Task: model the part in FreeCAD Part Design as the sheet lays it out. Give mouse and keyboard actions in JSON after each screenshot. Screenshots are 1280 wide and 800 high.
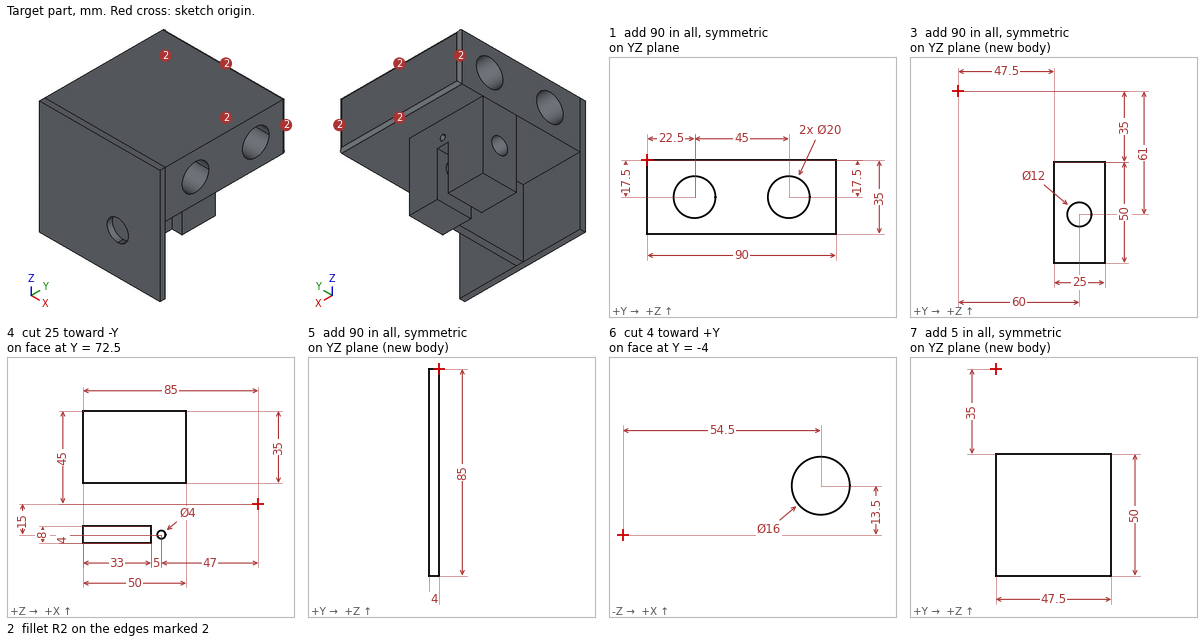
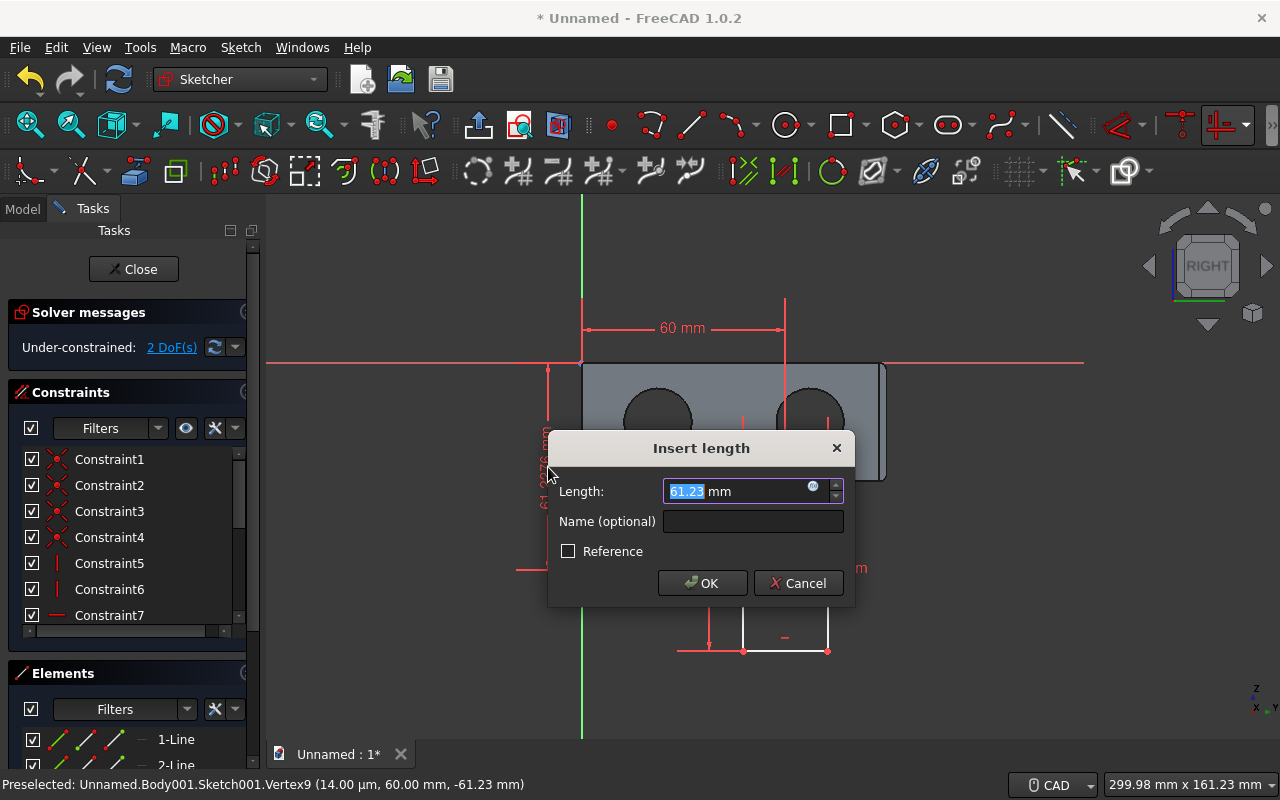
{"action": "type", "text": "61"}
{"action": "key", "text": "Return"}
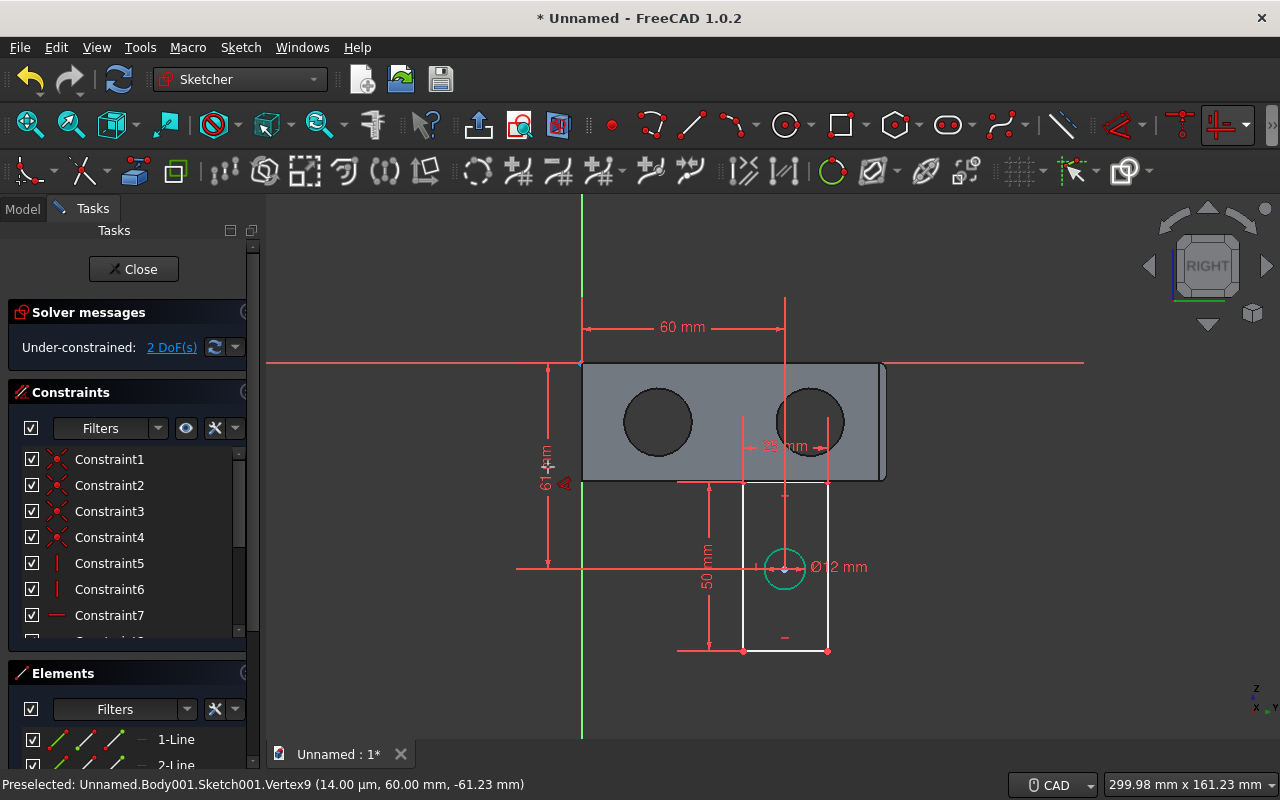
{"action": "left_click", "coordinate": [743, 482]}
{"action": "left_click", "coordinate": [548, 423]}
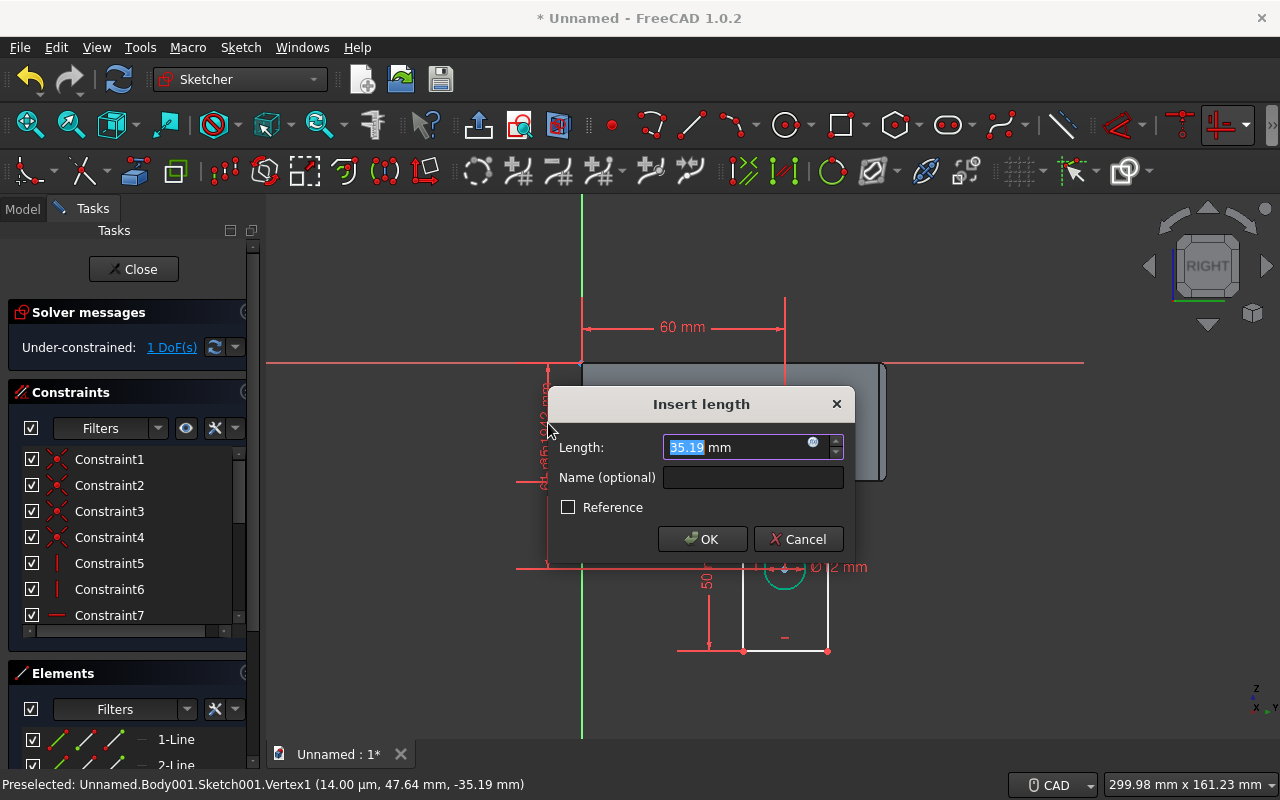
{"action": "type", "text": "35"}
{"action": "key", "text": "Return"}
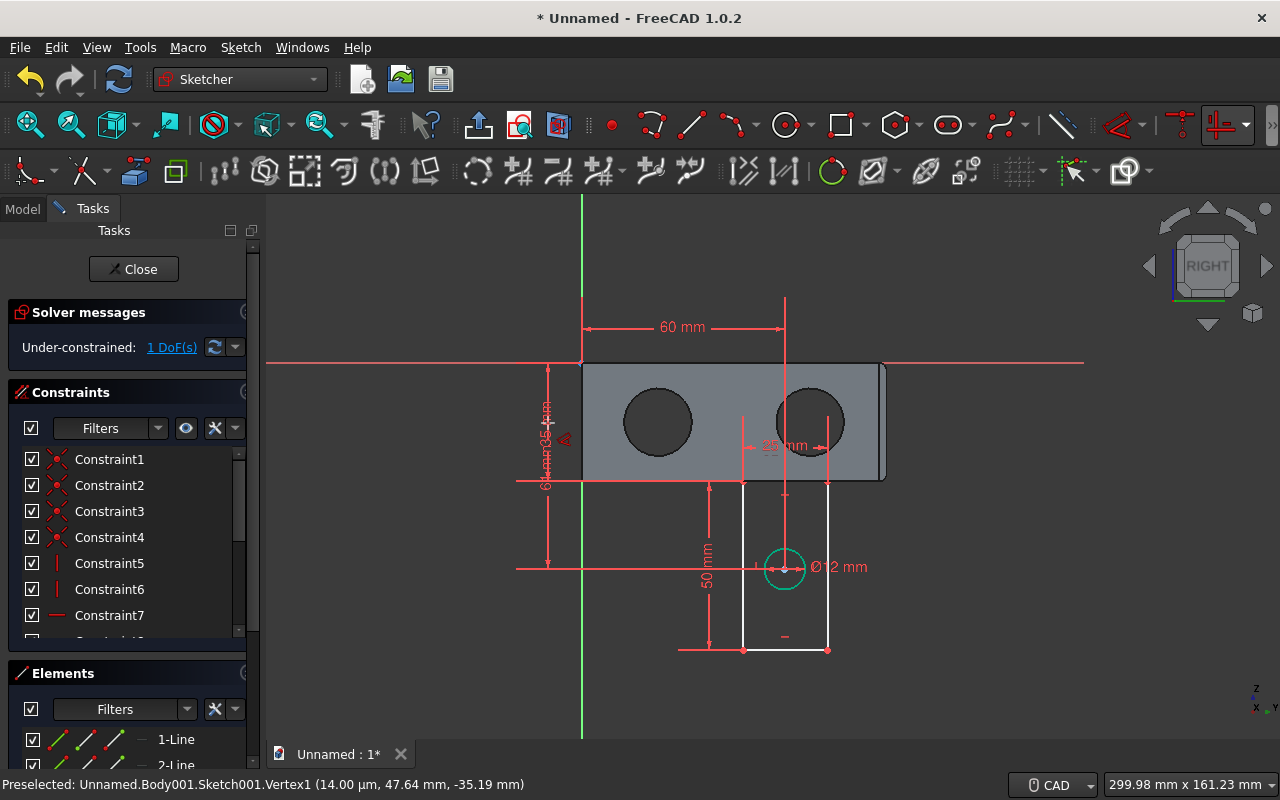
{"action": "left_click", "coordinate": [743, 481]}
{"action": "left_click", "coordinate": [606, 329]}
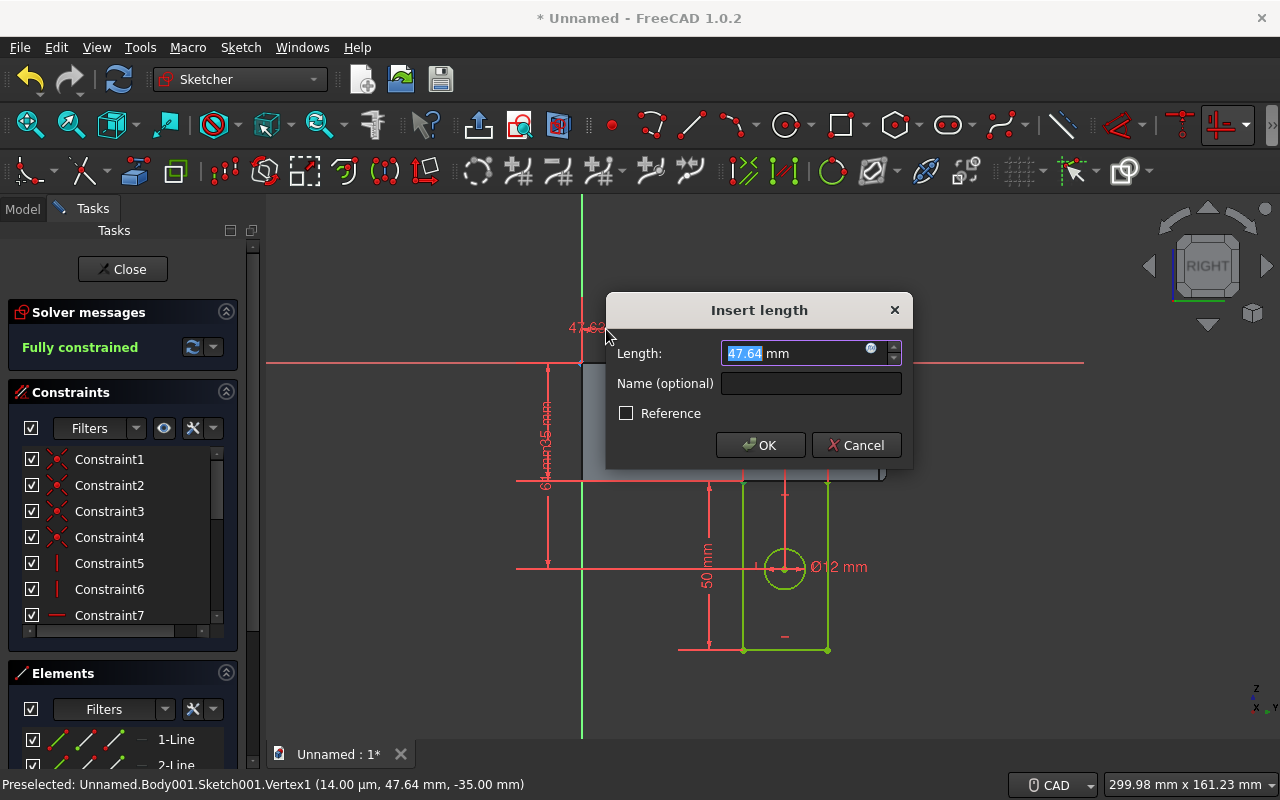
{"action": "type", "text": "47.5"}
{"action": "key", "text": "Return"}
{"action": "key", "text": "Escape"}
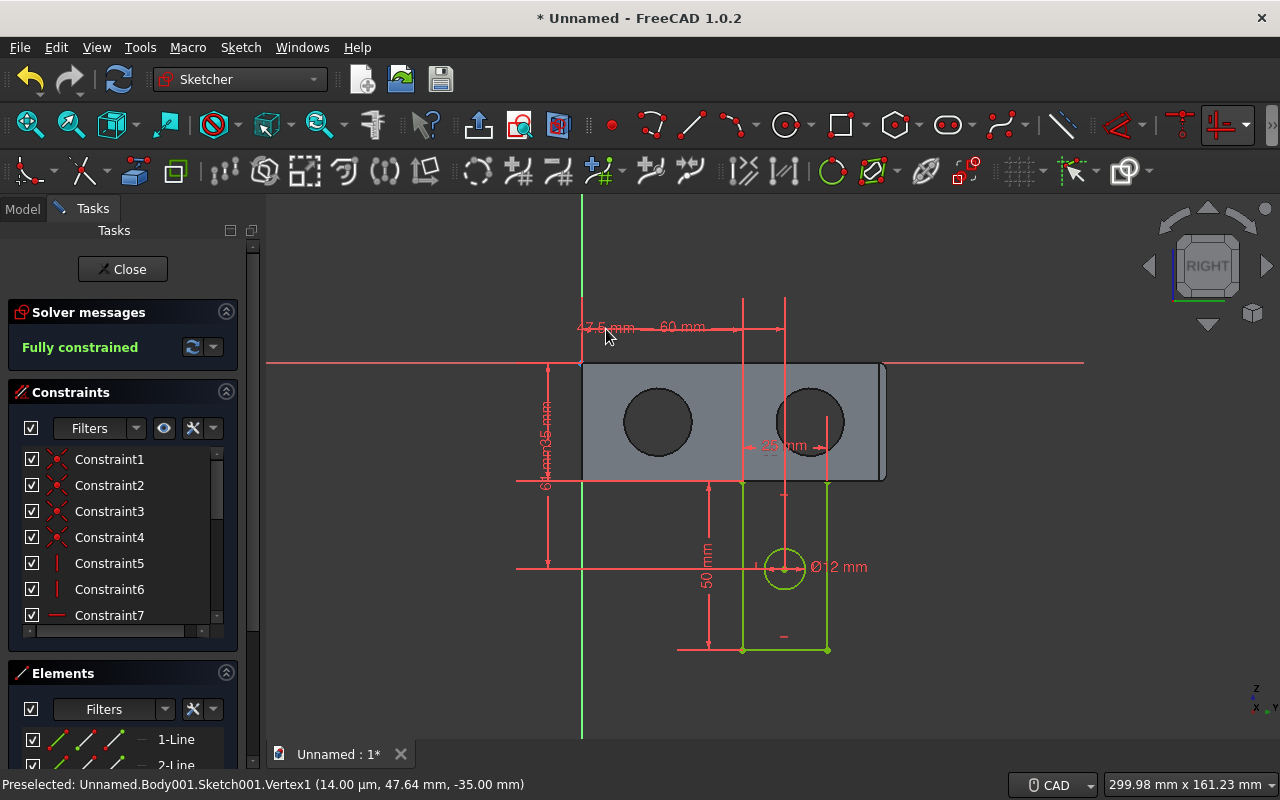
{"action": "left_click", "coordinate": [123, 269]}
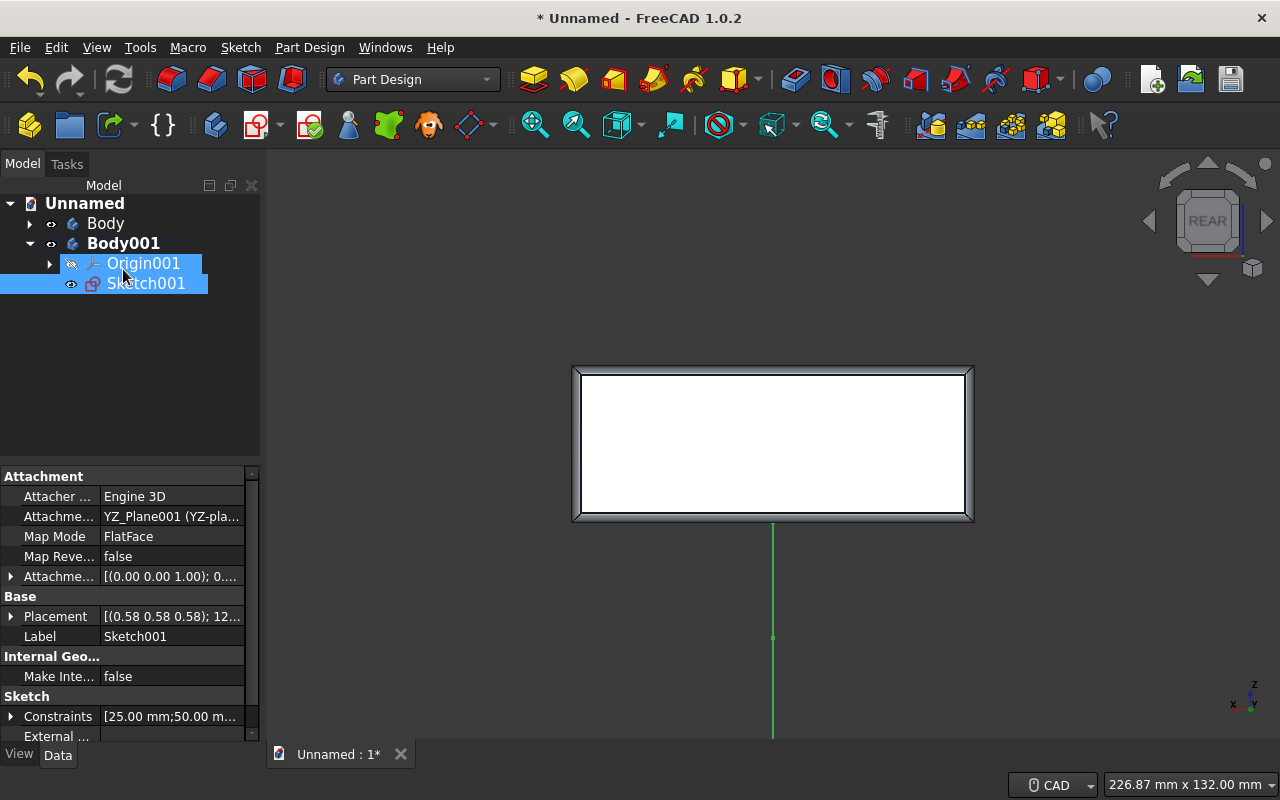
{"action": "left_click", "coordinate": [534, 80]}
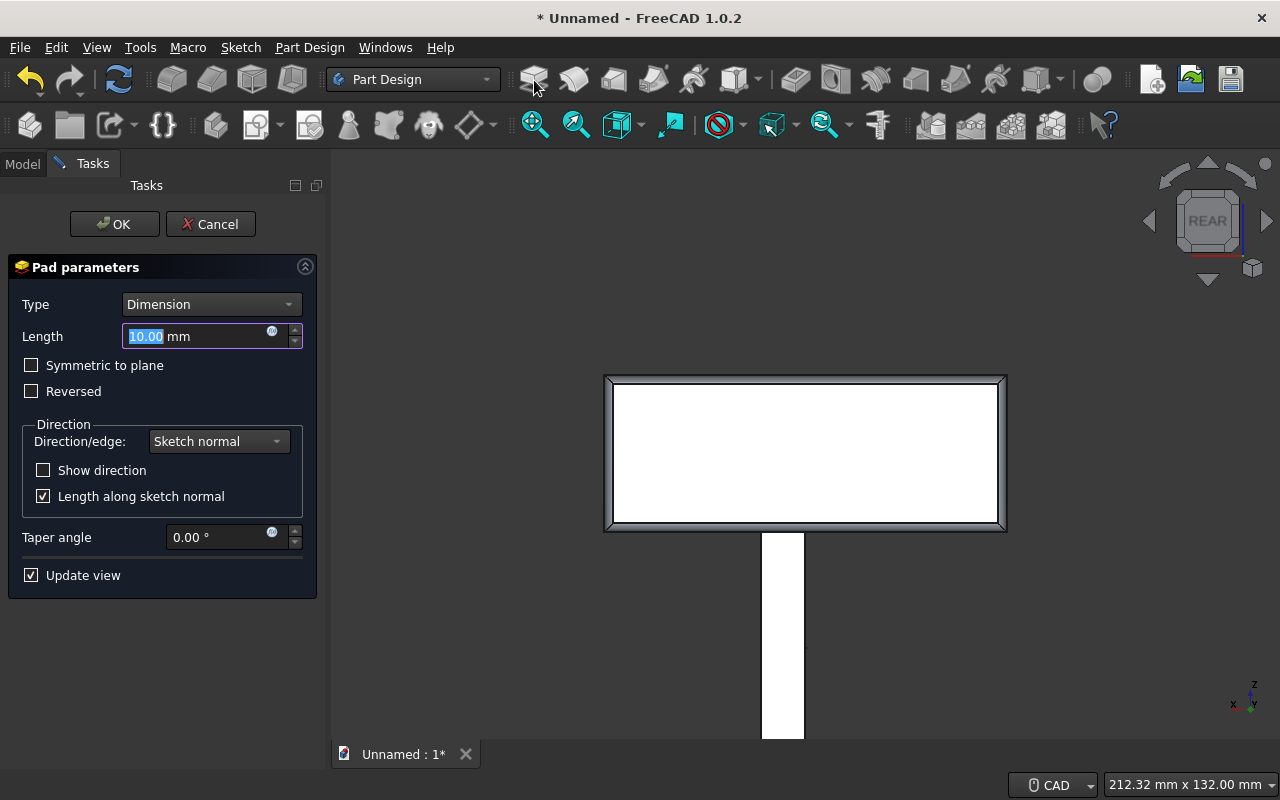
{"action": "type", "text": "90"}
{"action": "key", "text": "Tab"}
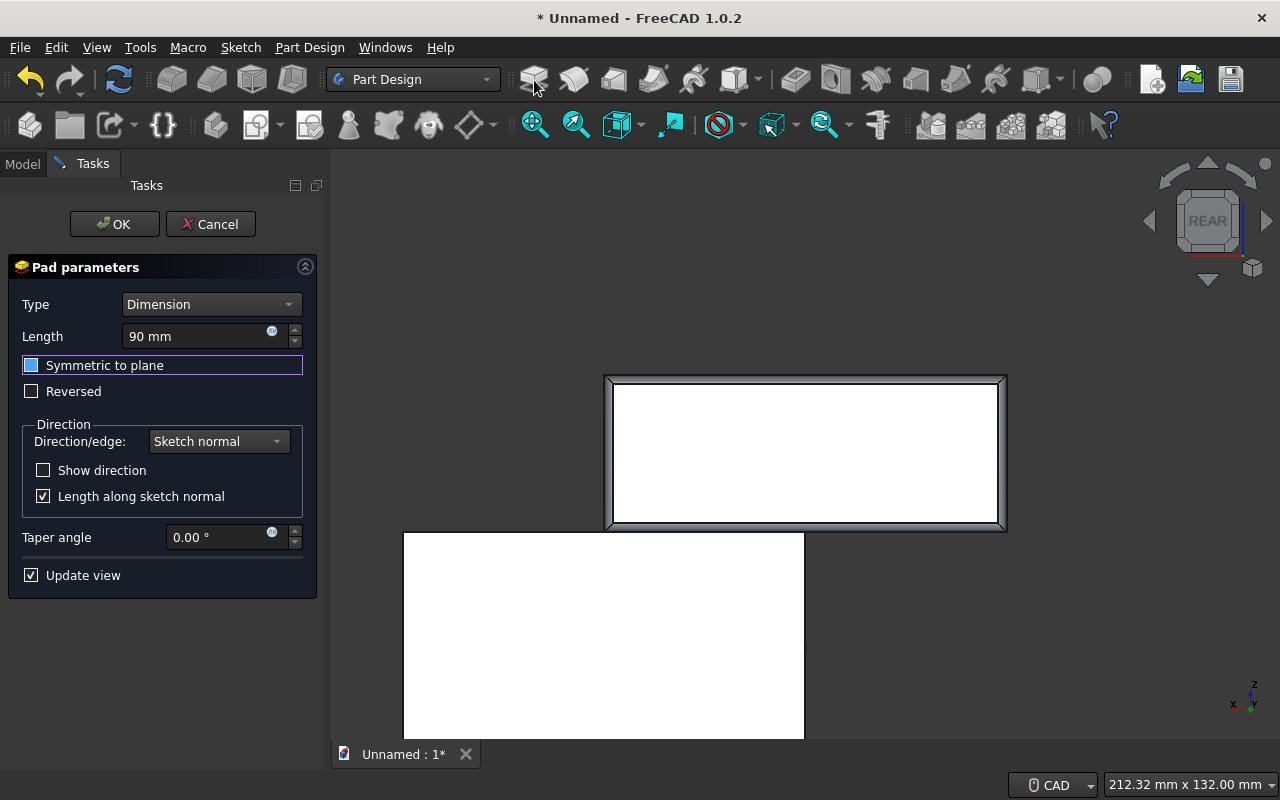
{"action": "left_click", "coordinate": [30, 365]}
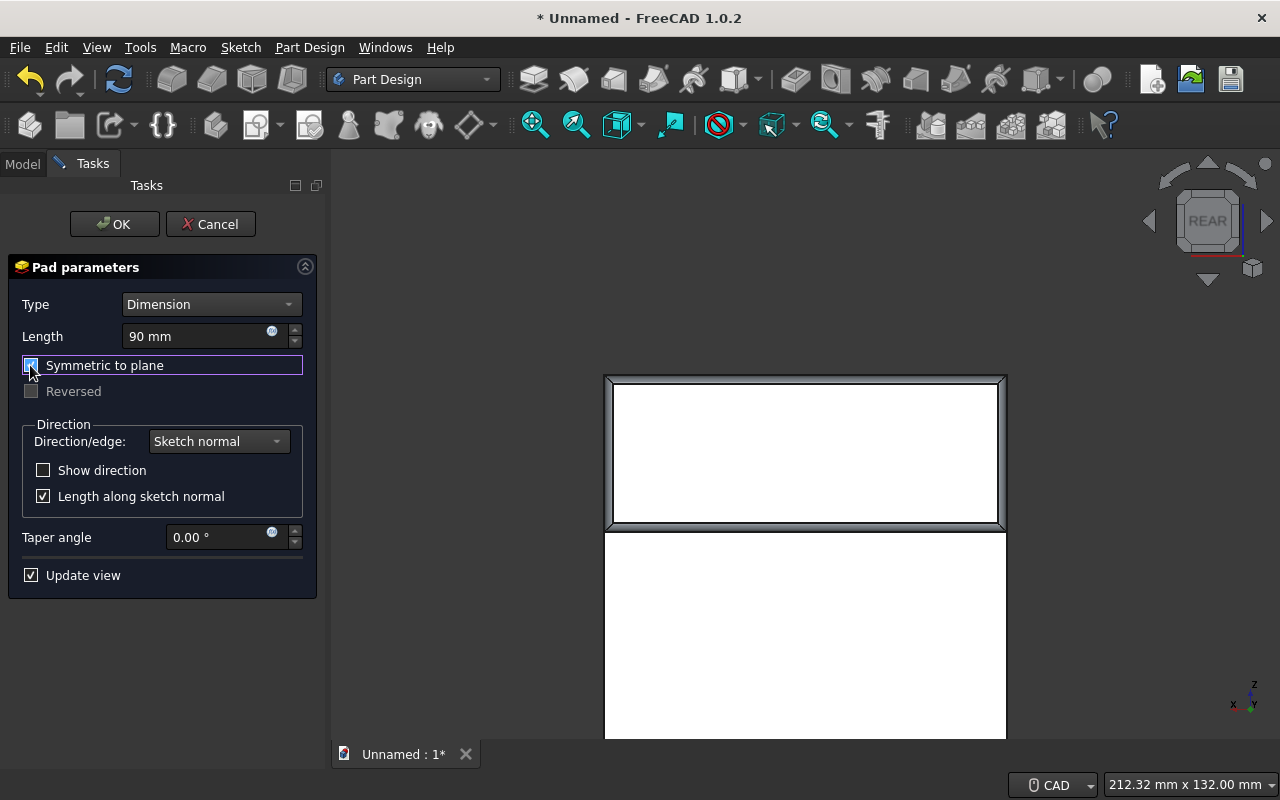
{"action": "left_click", "coordinate": [115, 224]}